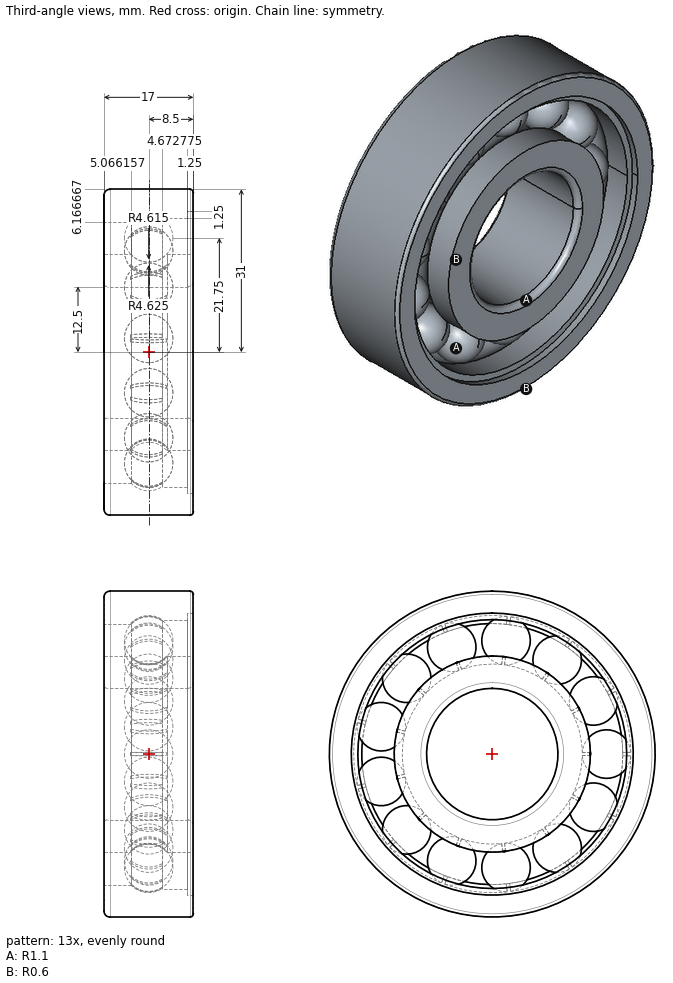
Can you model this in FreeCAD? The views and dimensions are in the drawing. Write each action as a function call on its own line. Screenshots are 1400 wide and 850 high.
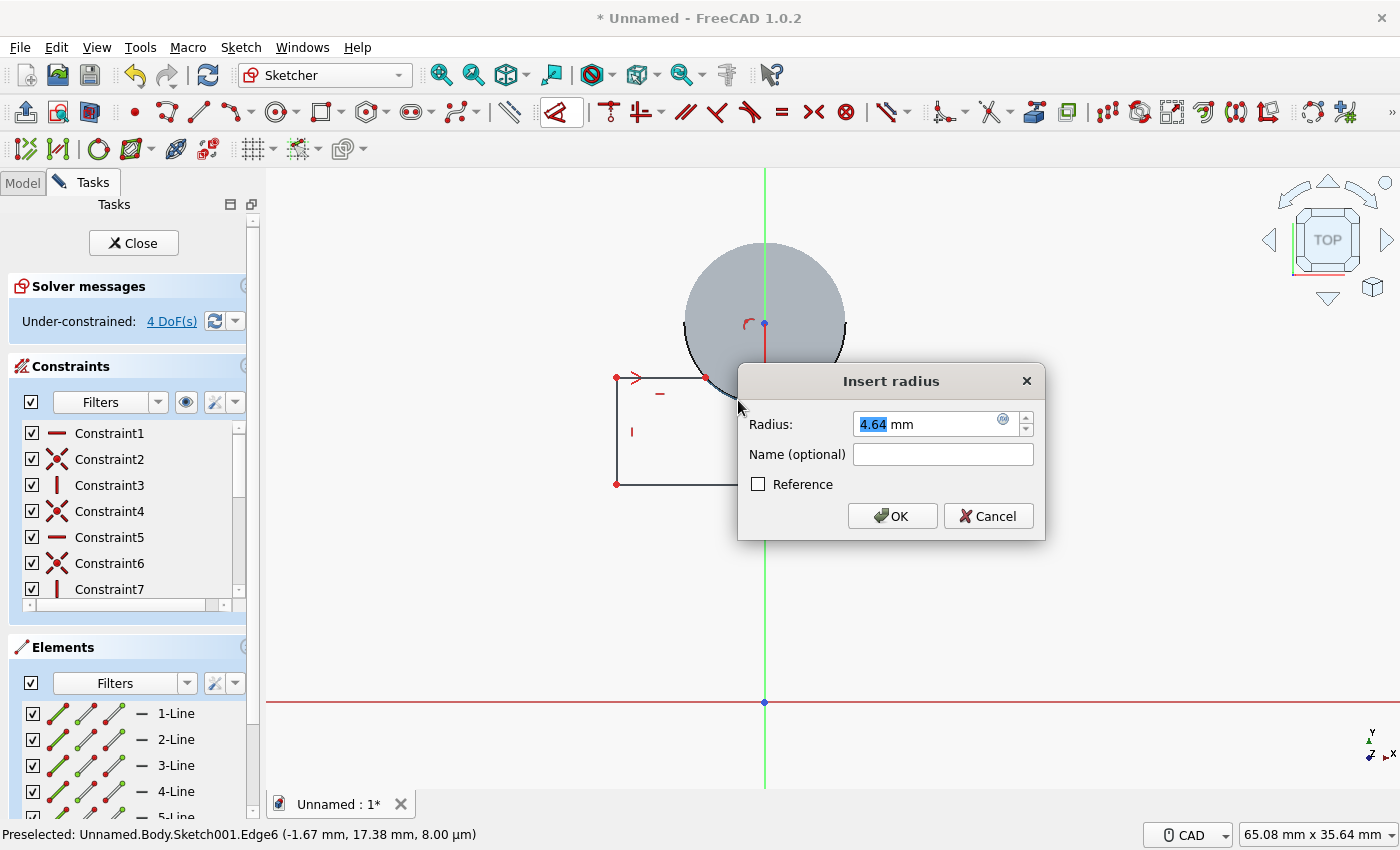
text(4.615)
key(Return)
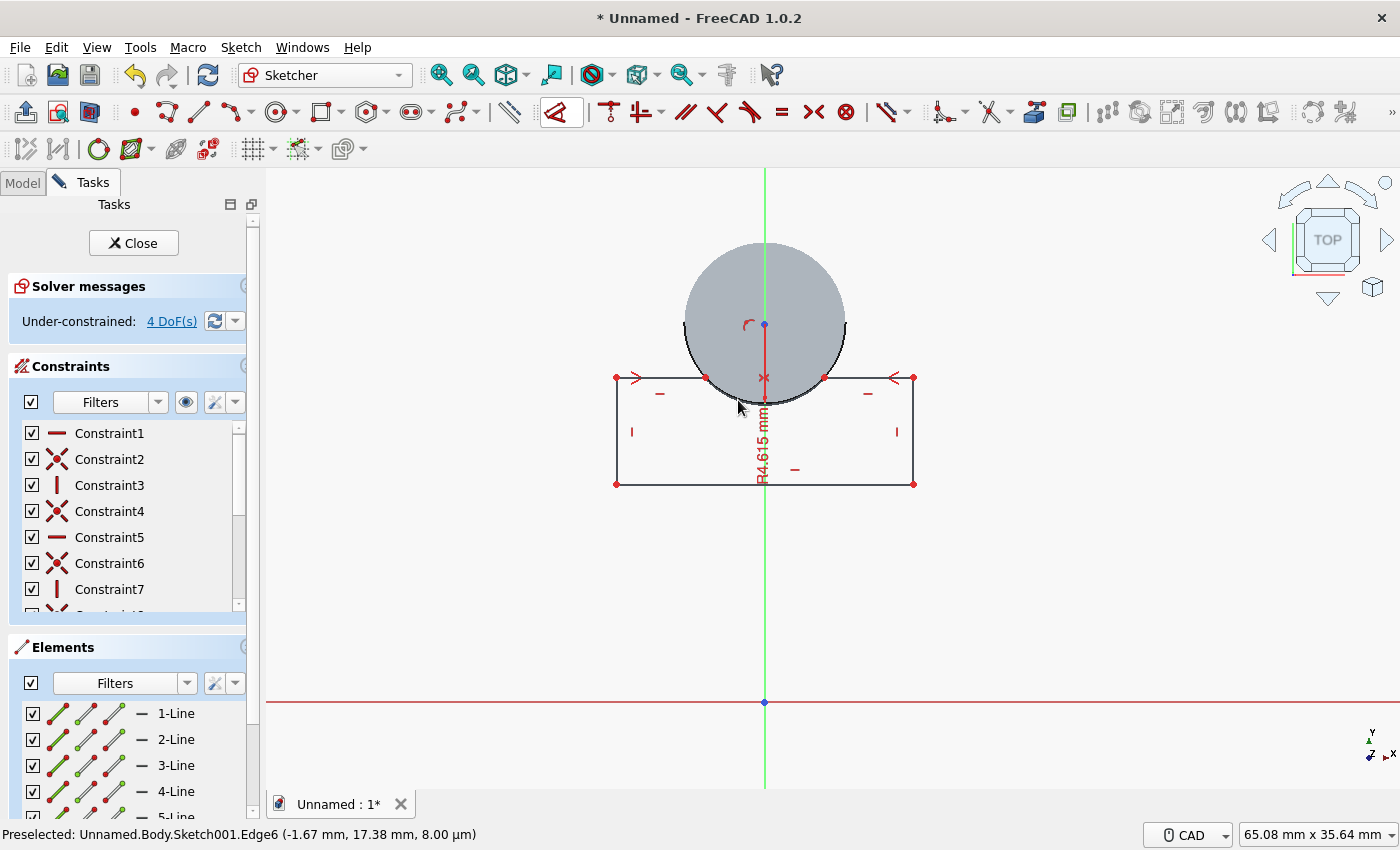
click(706, 485)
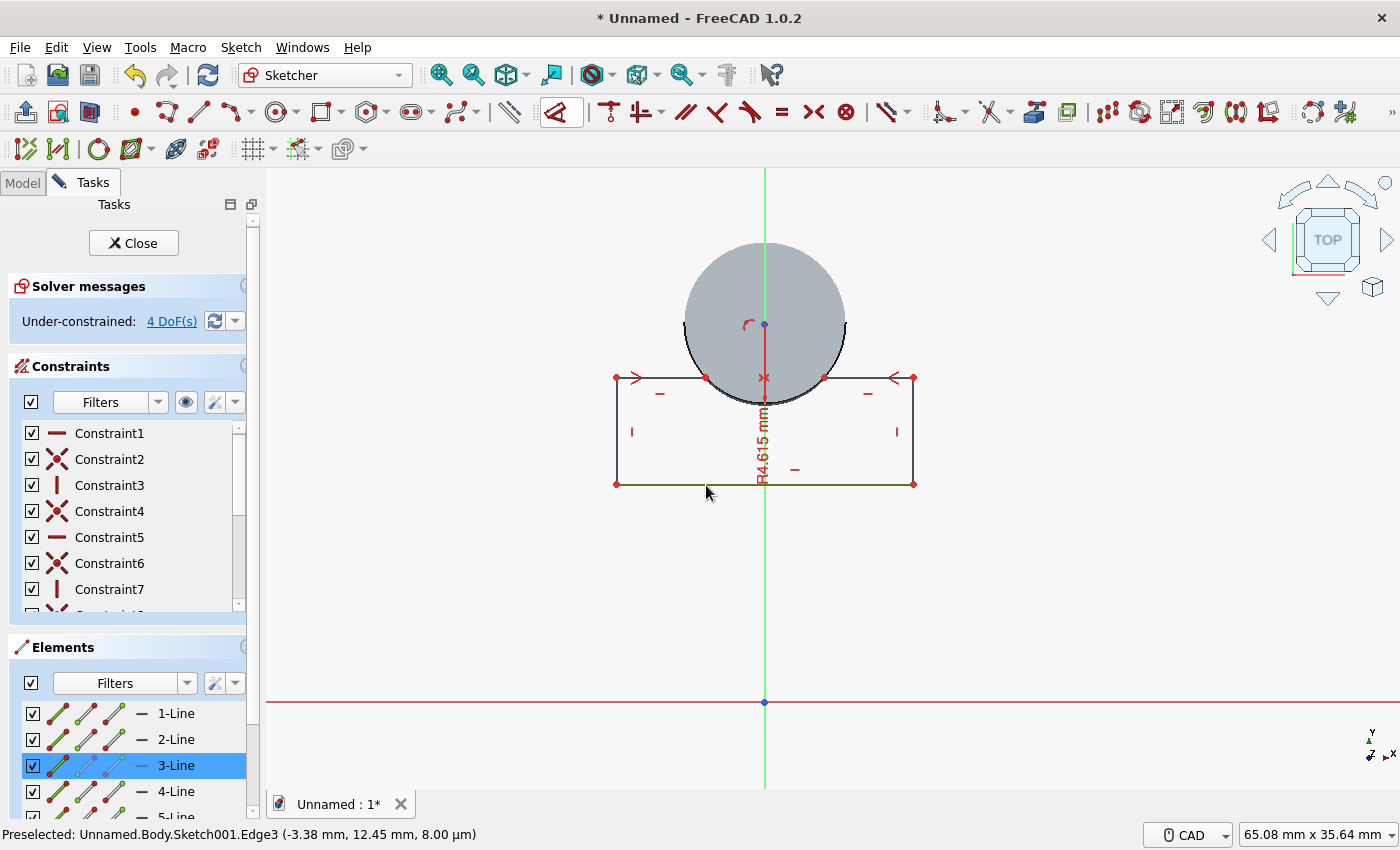
click(578, 112)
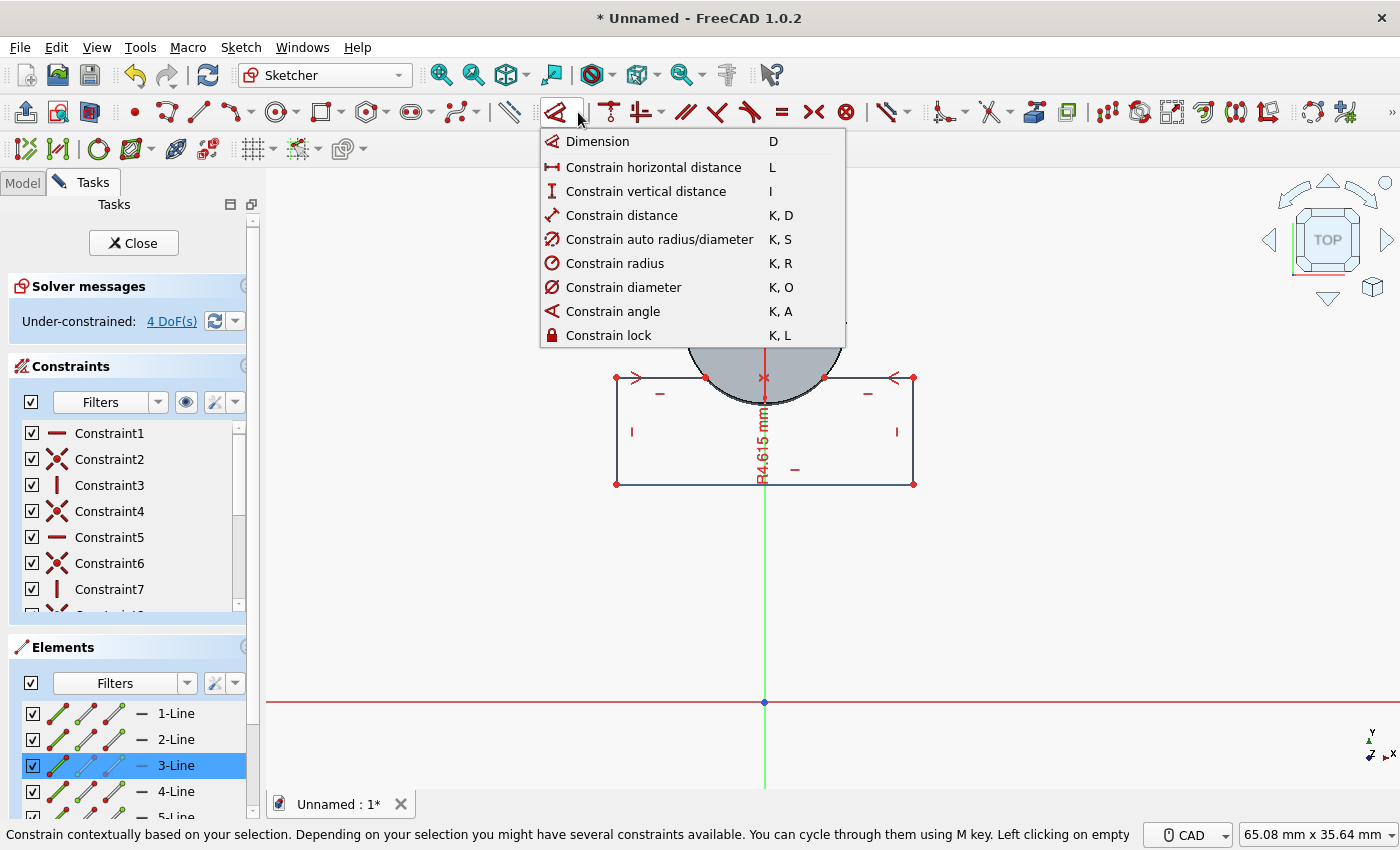
click(693, 167)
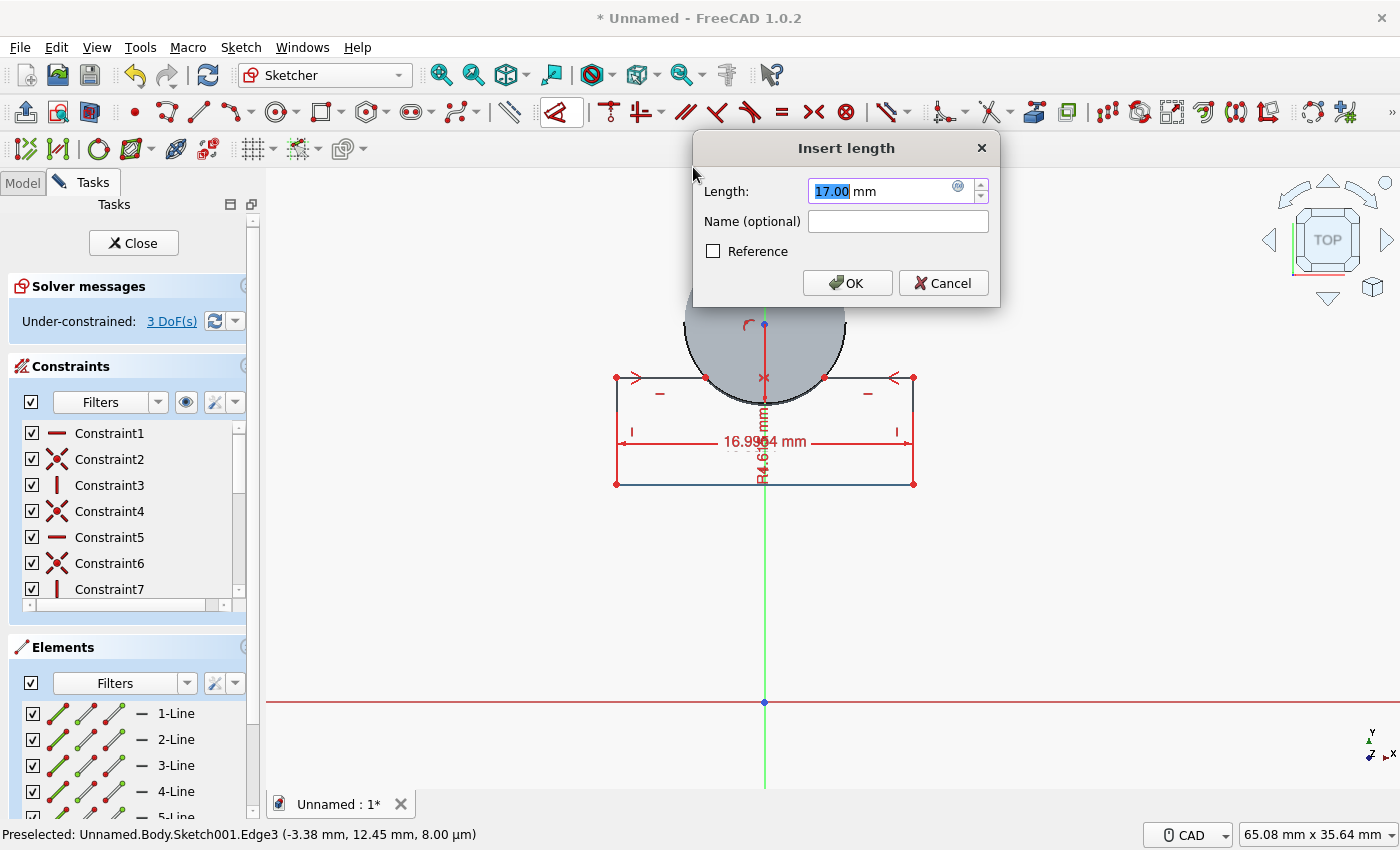
text(17)
key(Return)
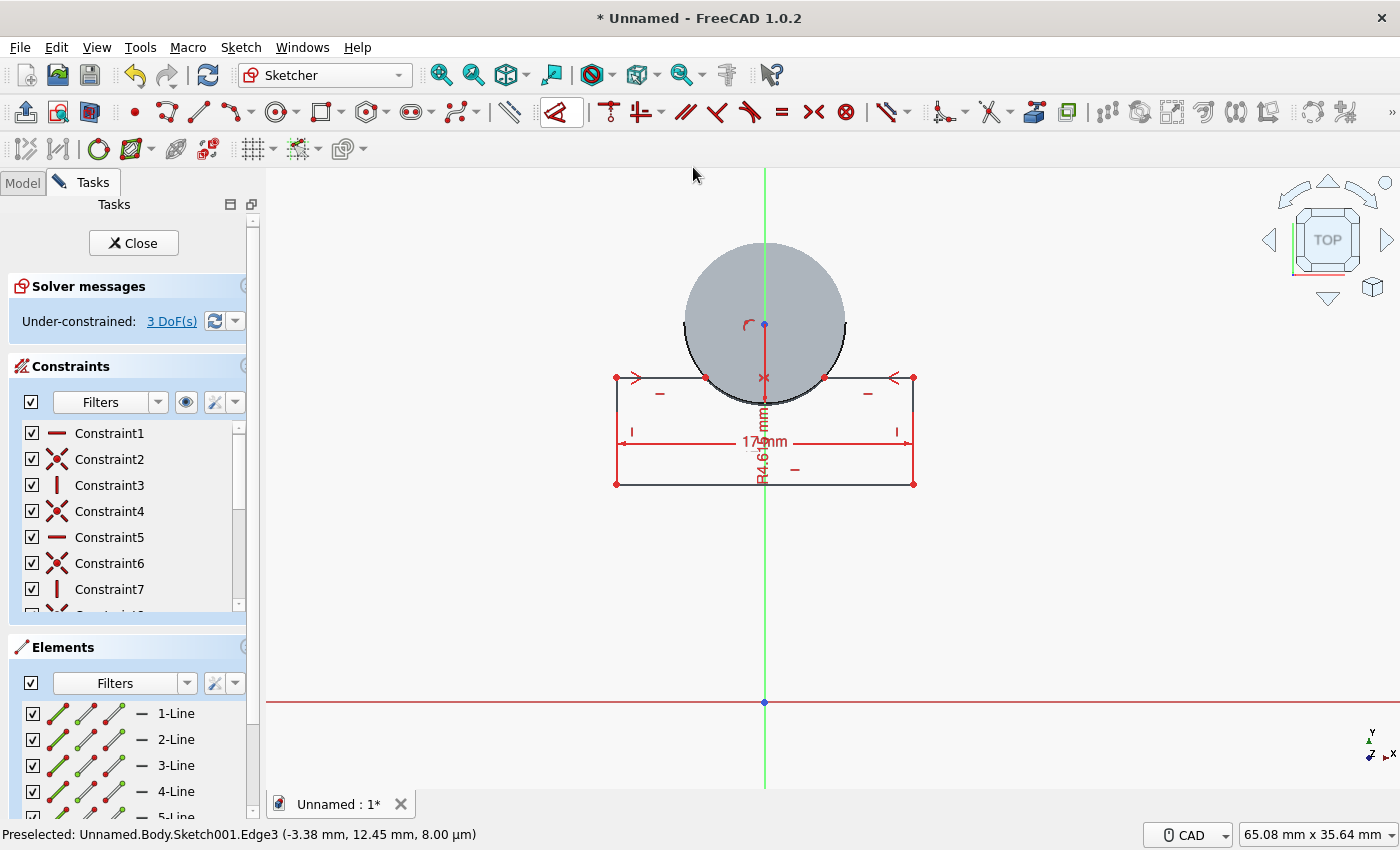
click(617, 485)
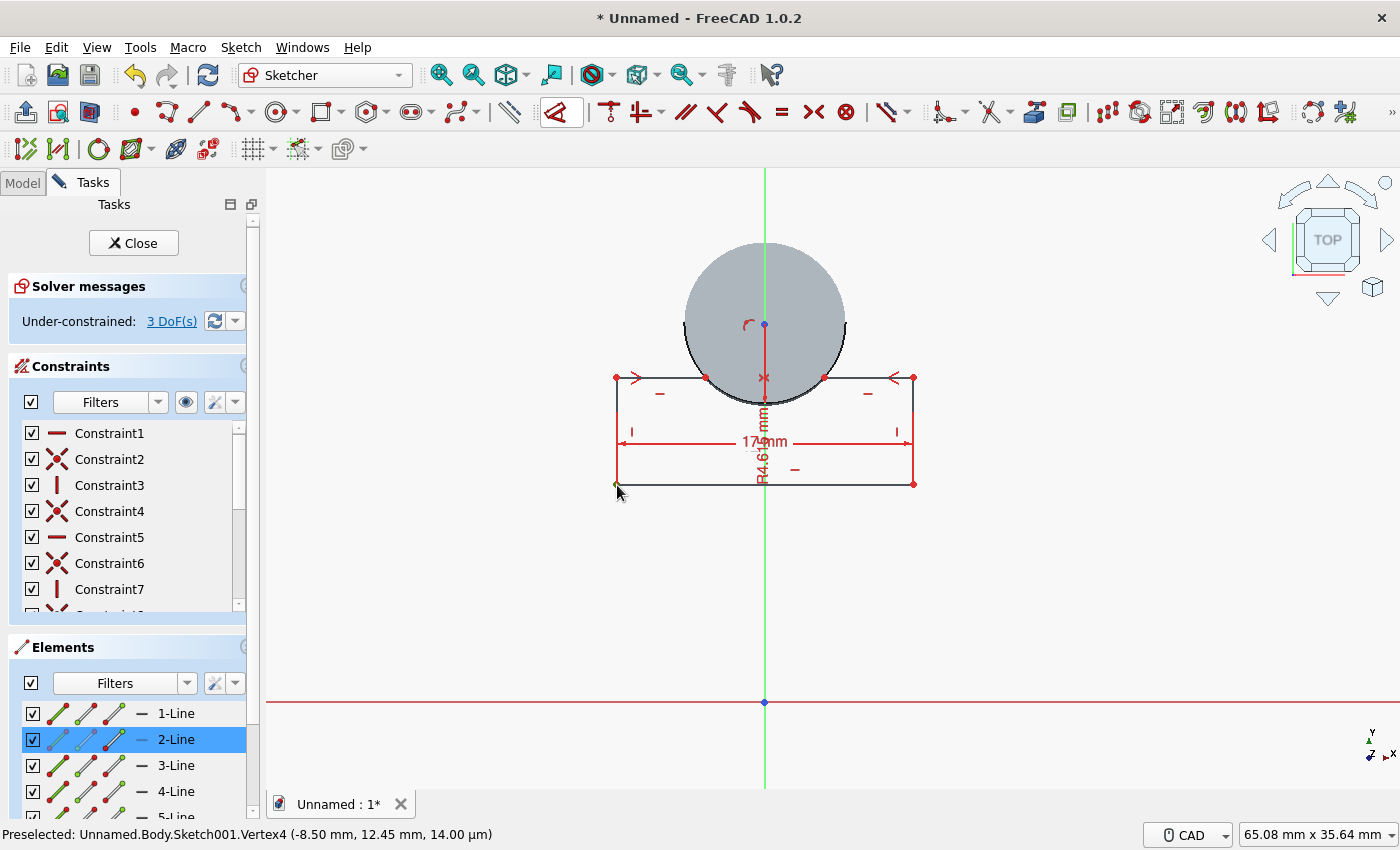
key(i)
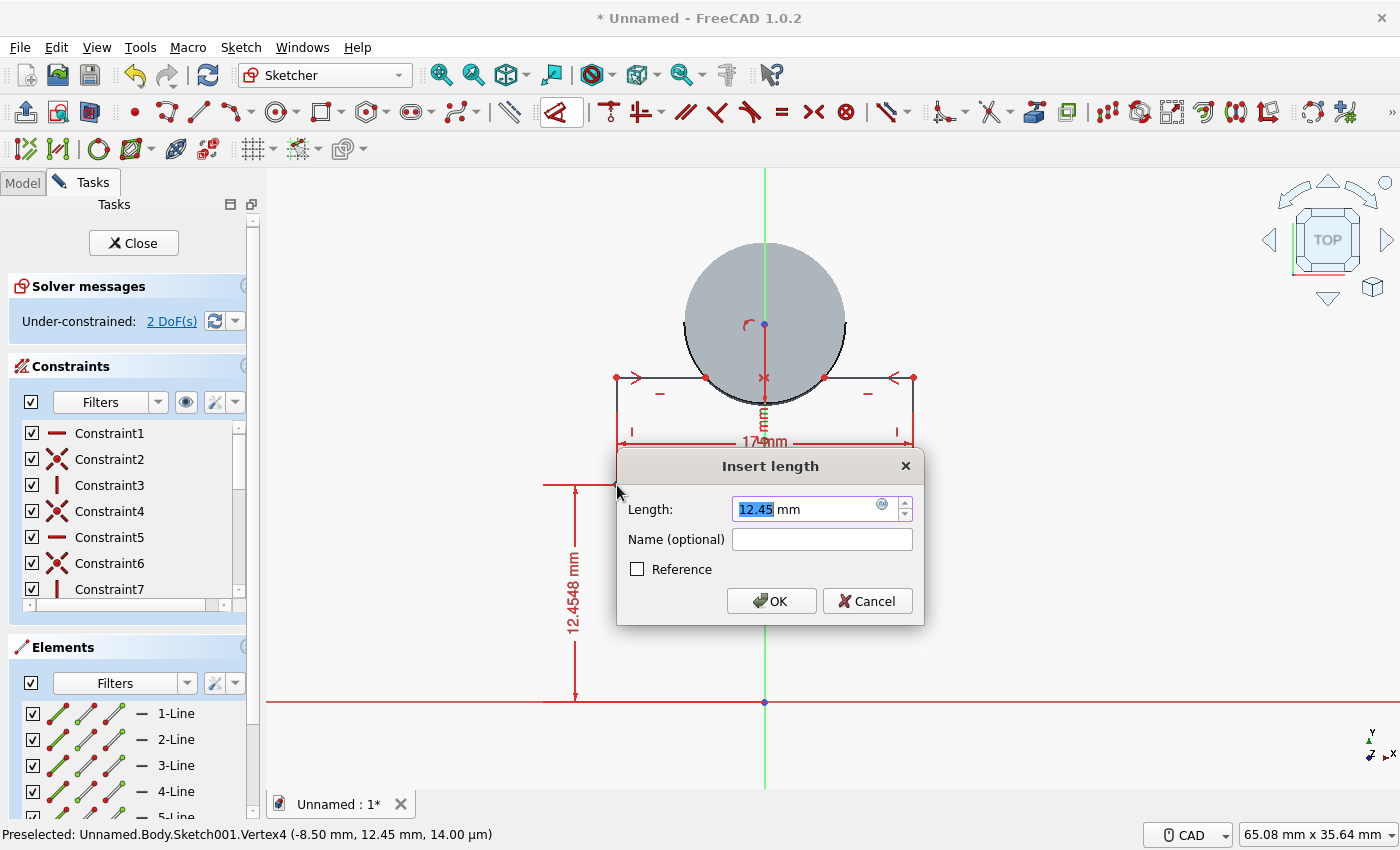
text(12.5)
key(Return)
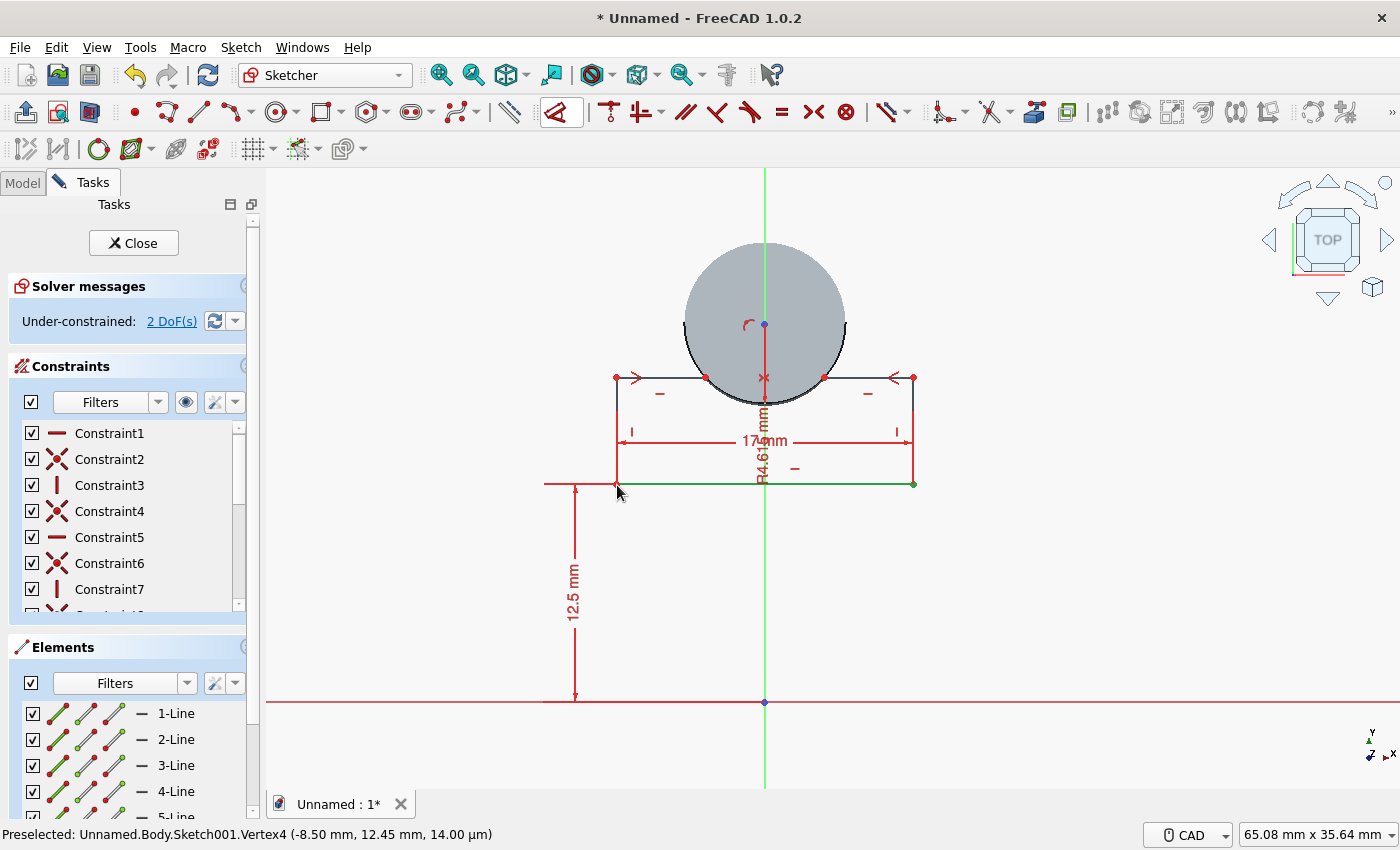
click(765, 324)